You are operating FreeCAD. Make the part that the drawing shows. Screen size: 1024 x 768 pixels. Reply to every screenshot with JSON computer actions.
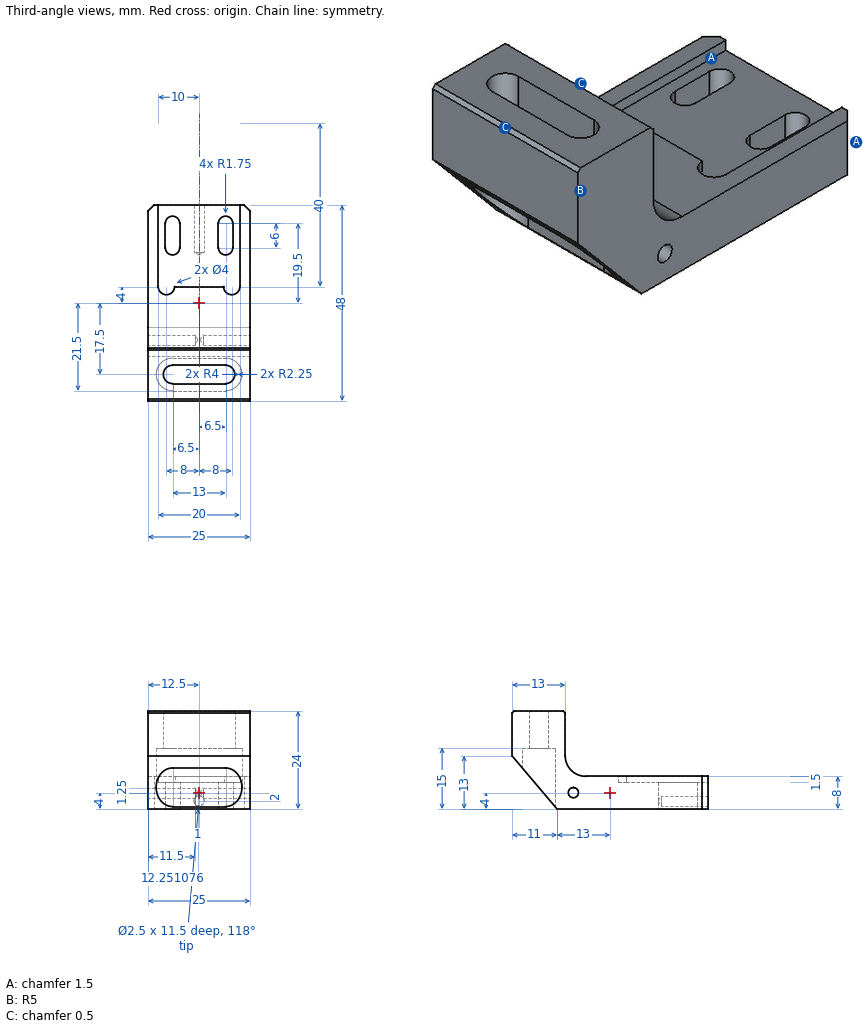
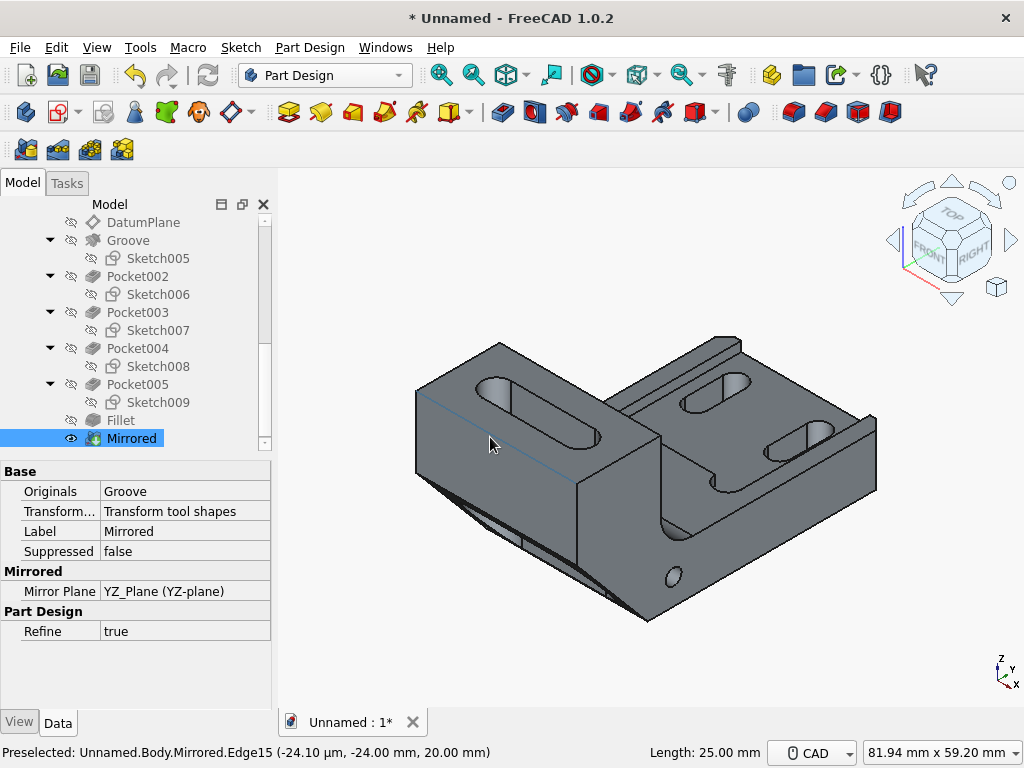
{"action": "key", "text": "2"}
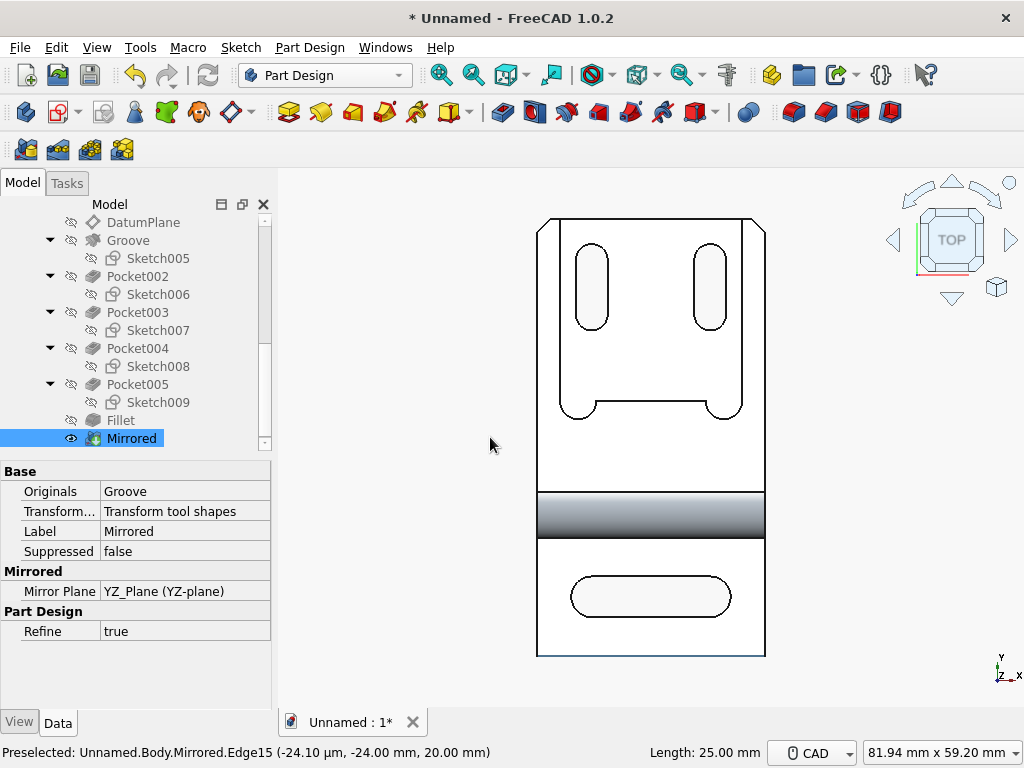
{"action": "left_click", "coordinate": [651, 537], "text": "ctrl"}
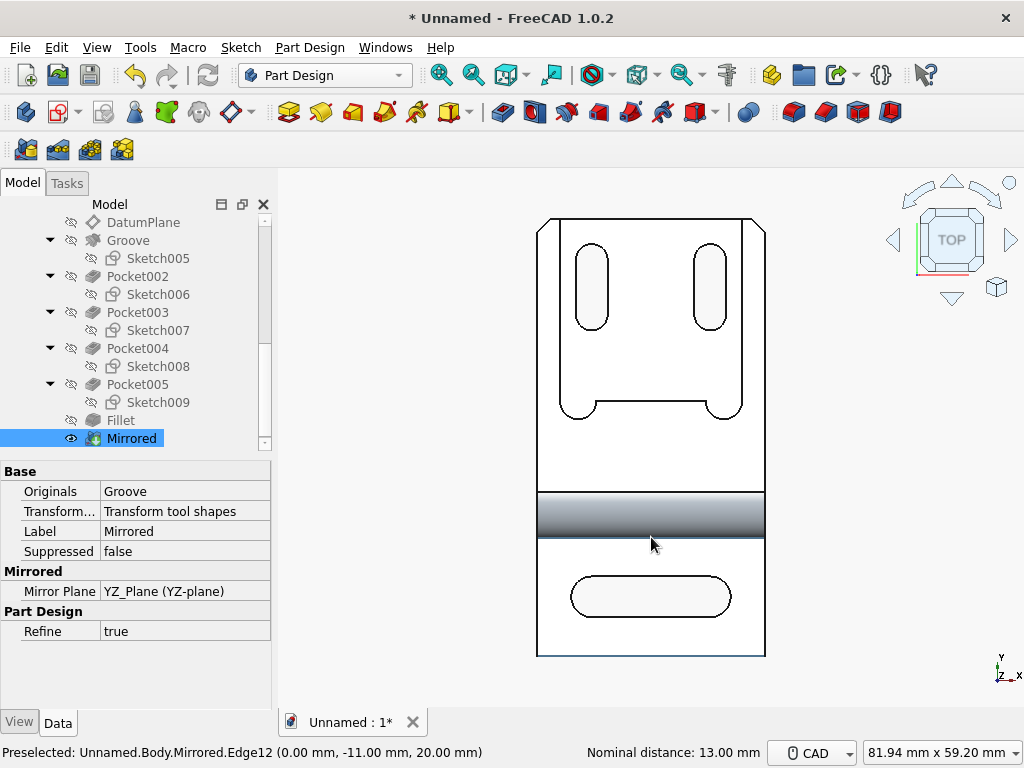
{"action": "left_click", "coordinate": [826, 112]}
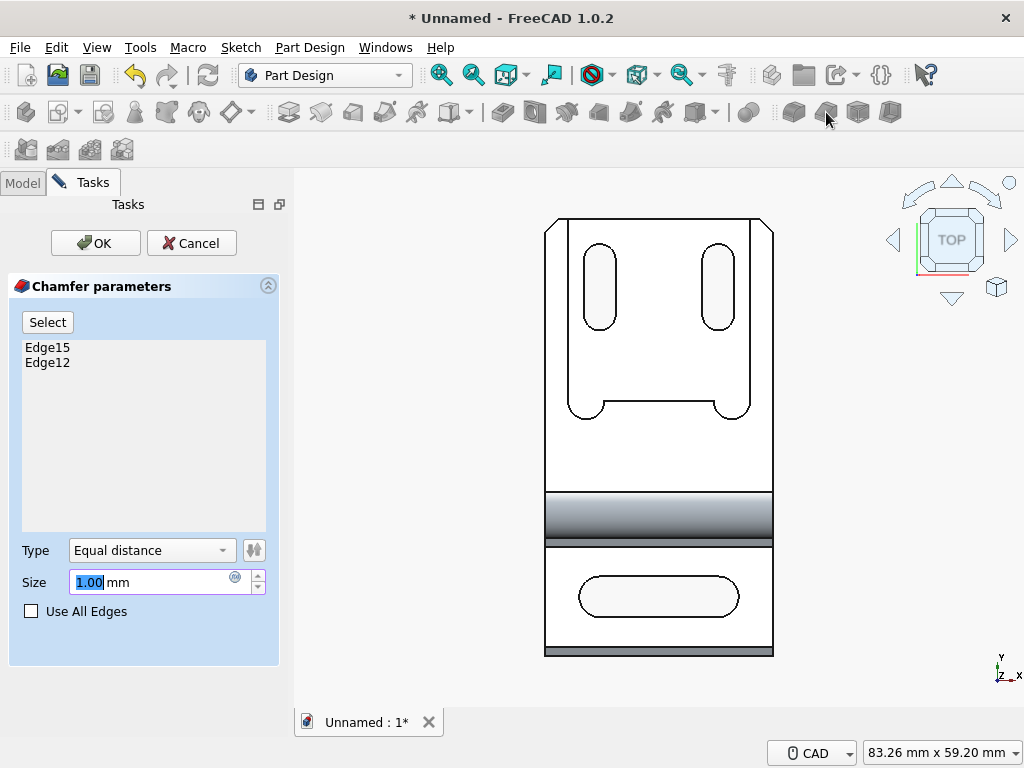
{"action": "type", "text": "0.5"}
{"action": "key", "text": "Tab"}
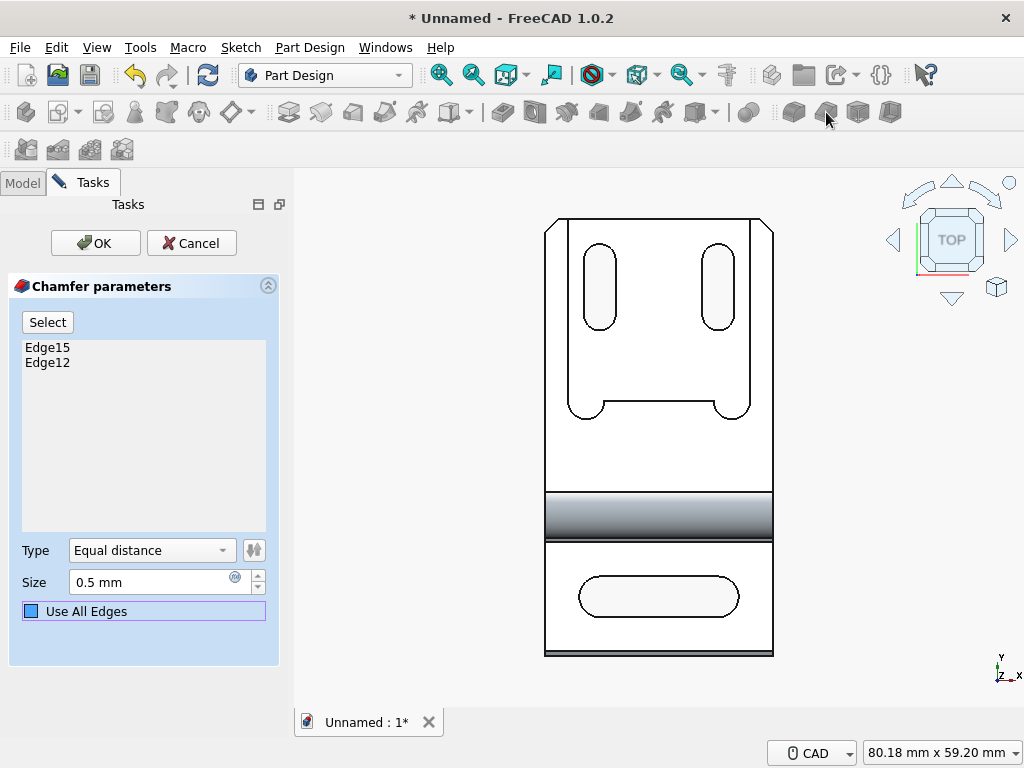
{"action": "left_click", "coordinate": [96, 243]}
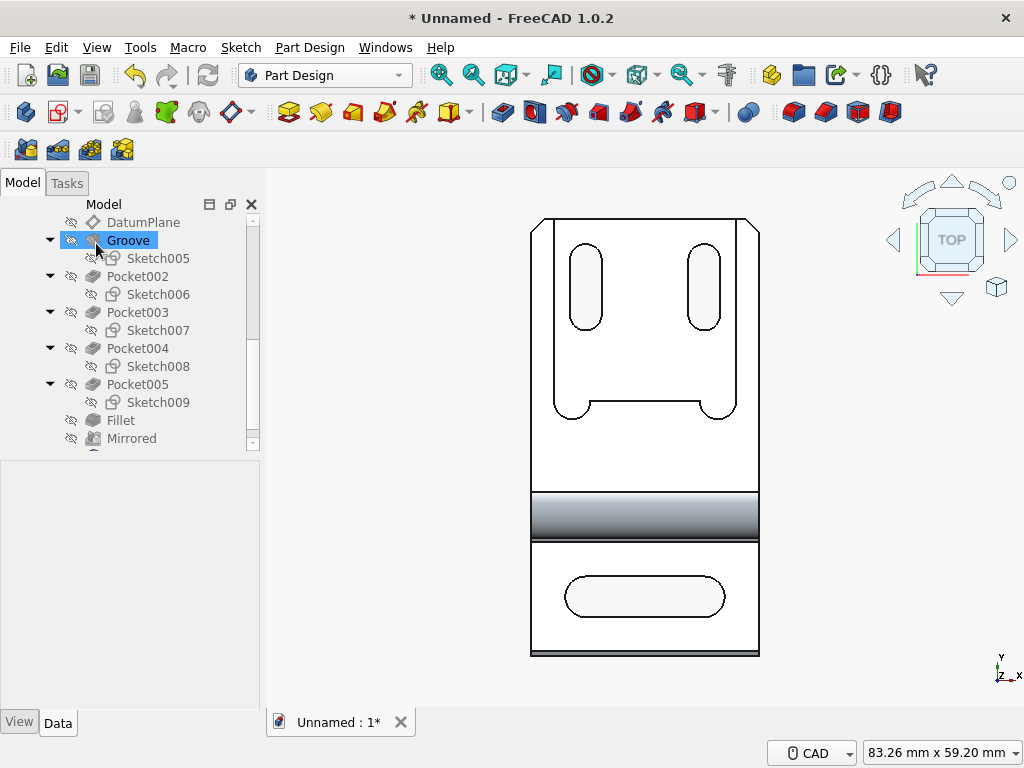
{"action": "key", "text": "0"}